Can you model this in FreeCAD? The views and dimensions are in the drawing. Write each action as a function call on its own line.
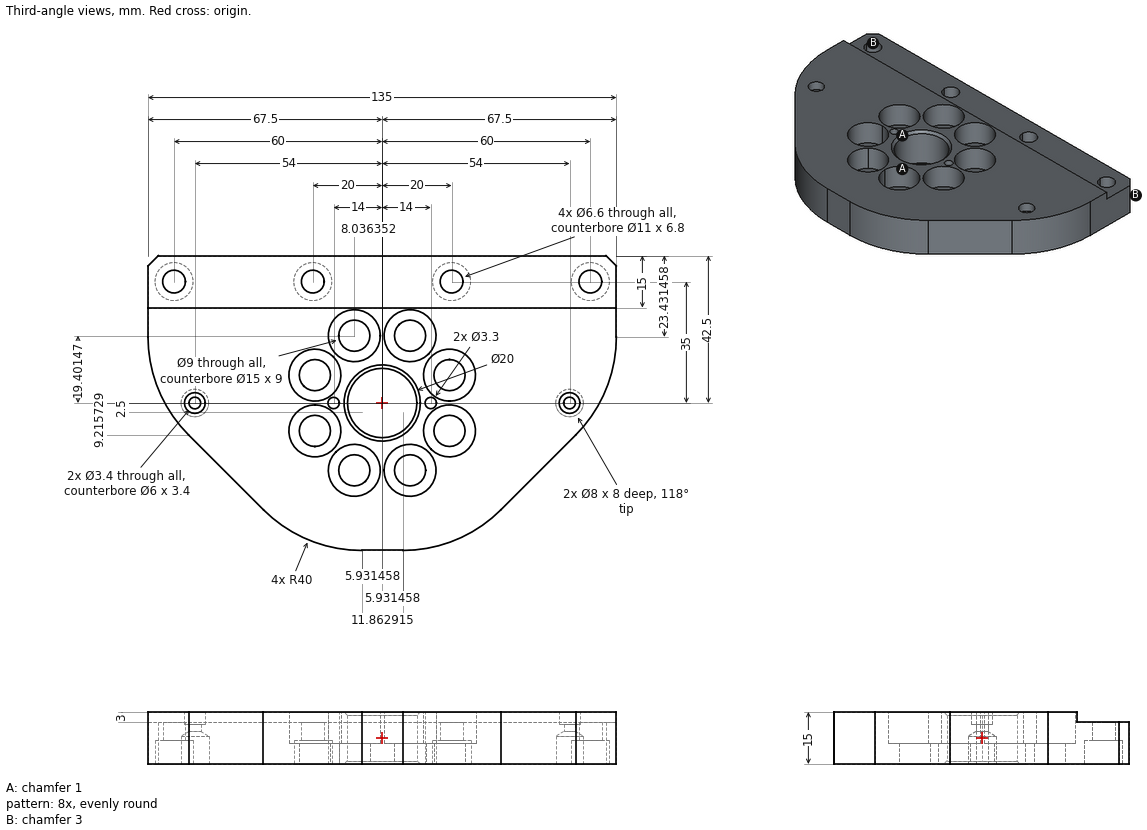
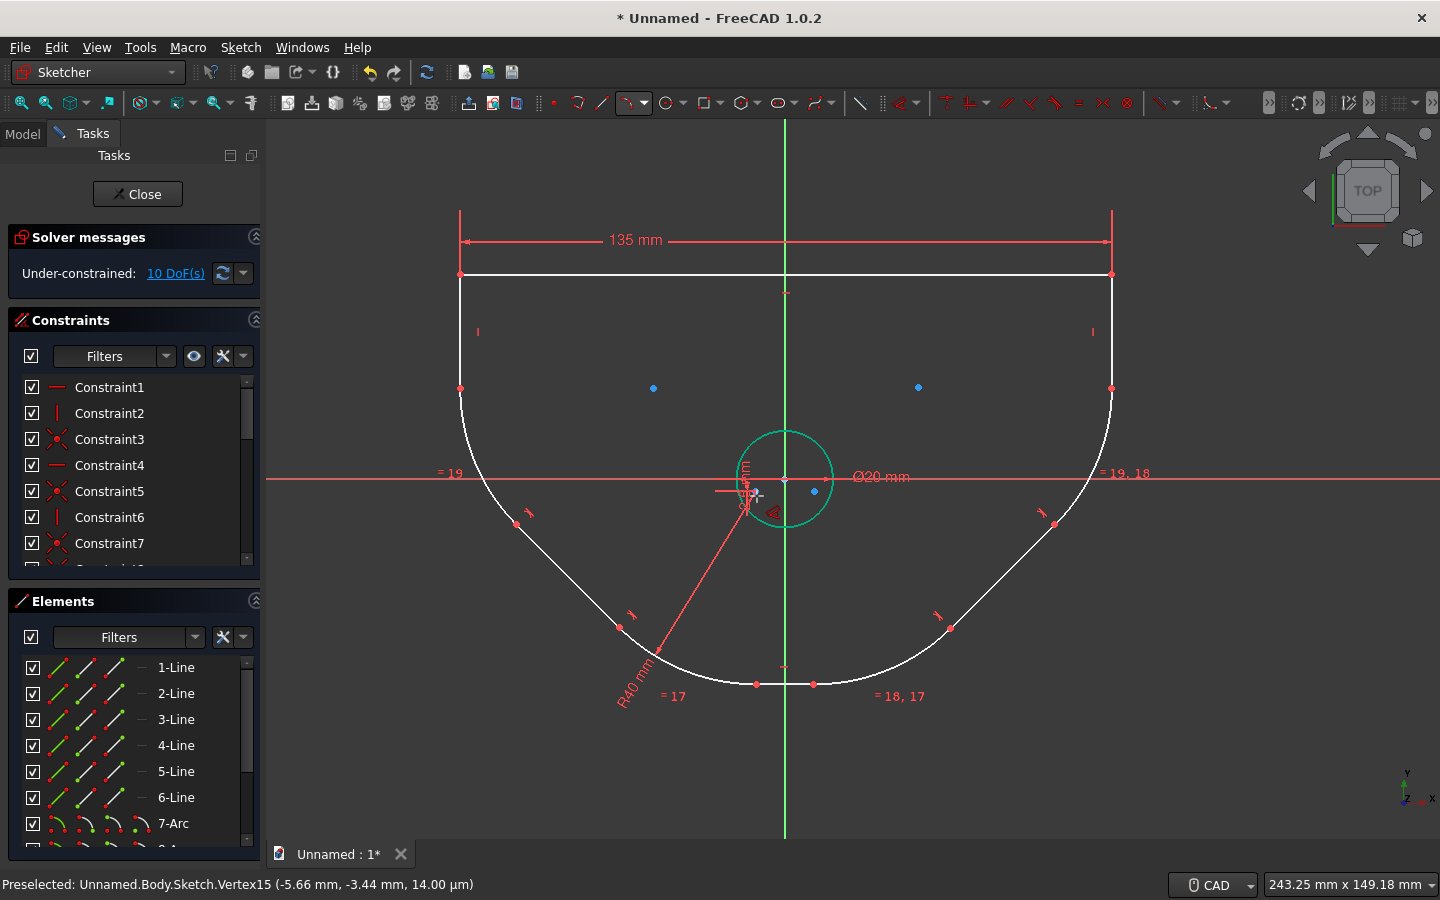
click(1112, 388)
click(948, 354)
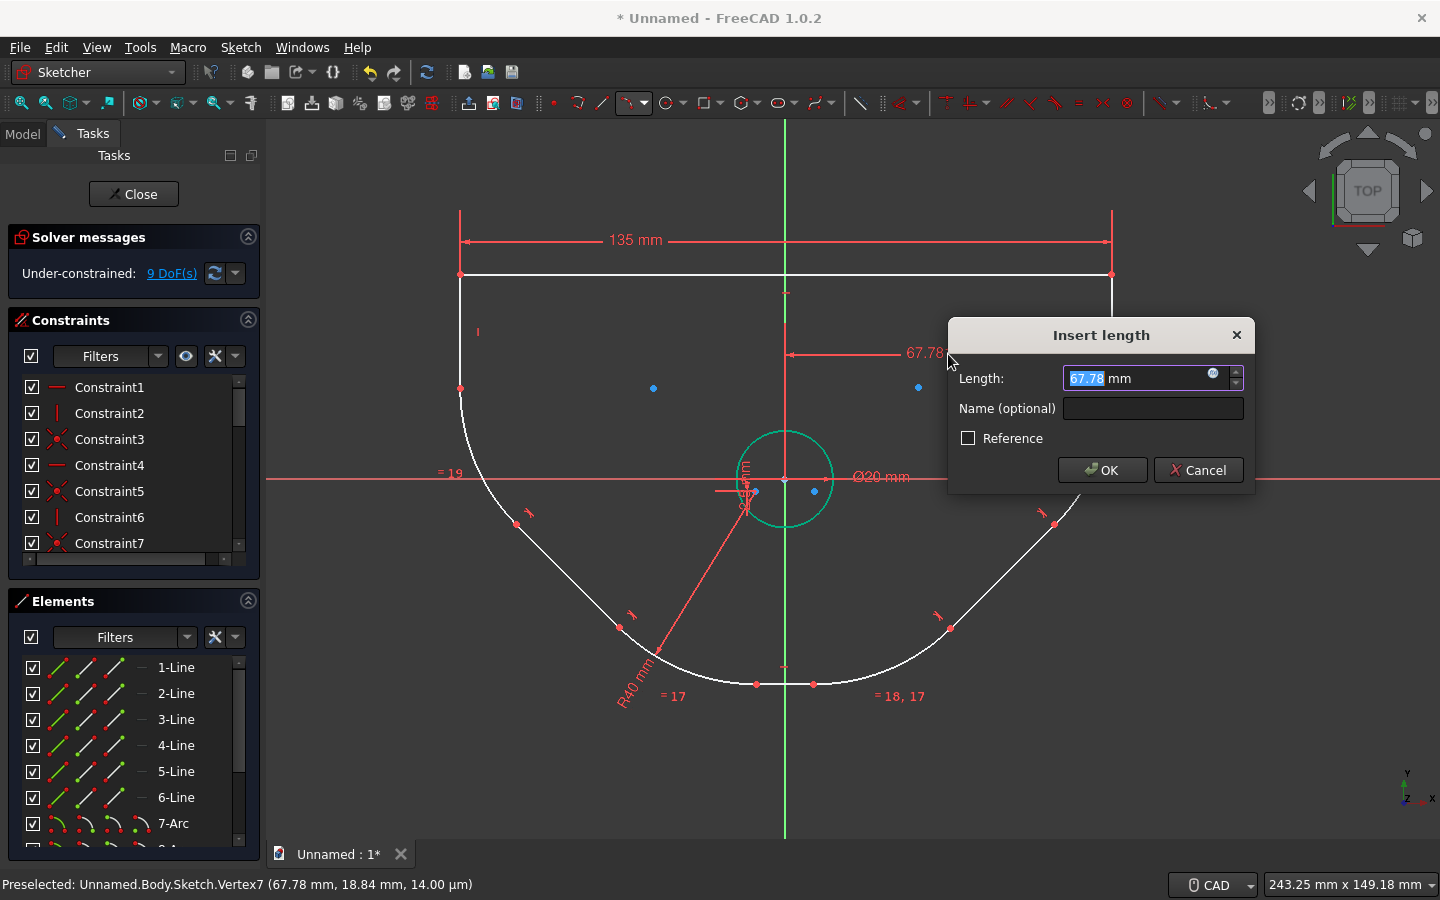
text(67.5)
key(Return)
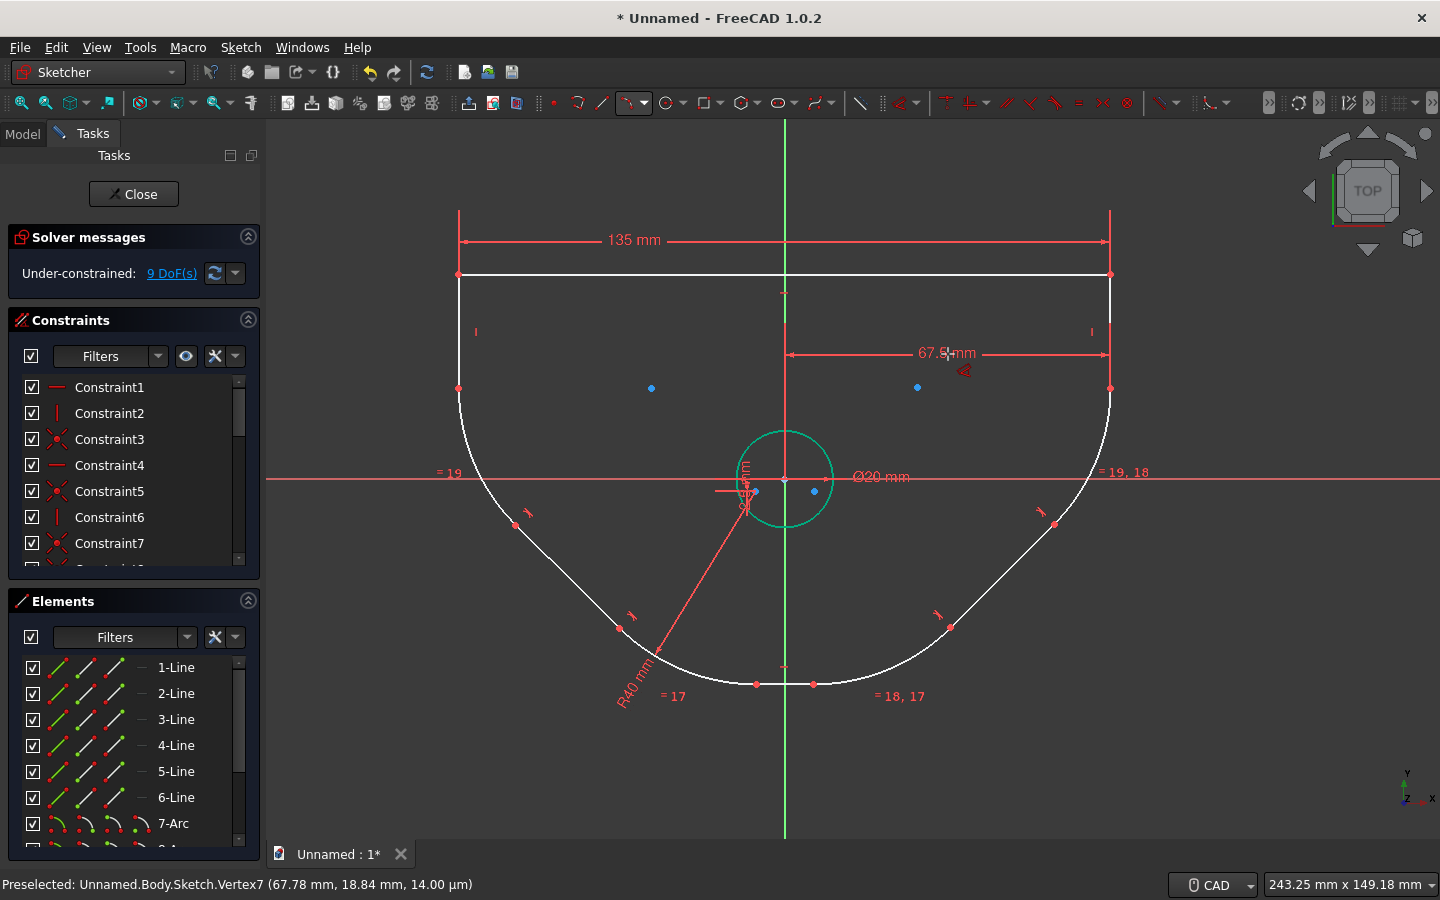
click(1110, 275)
click(1144, 377)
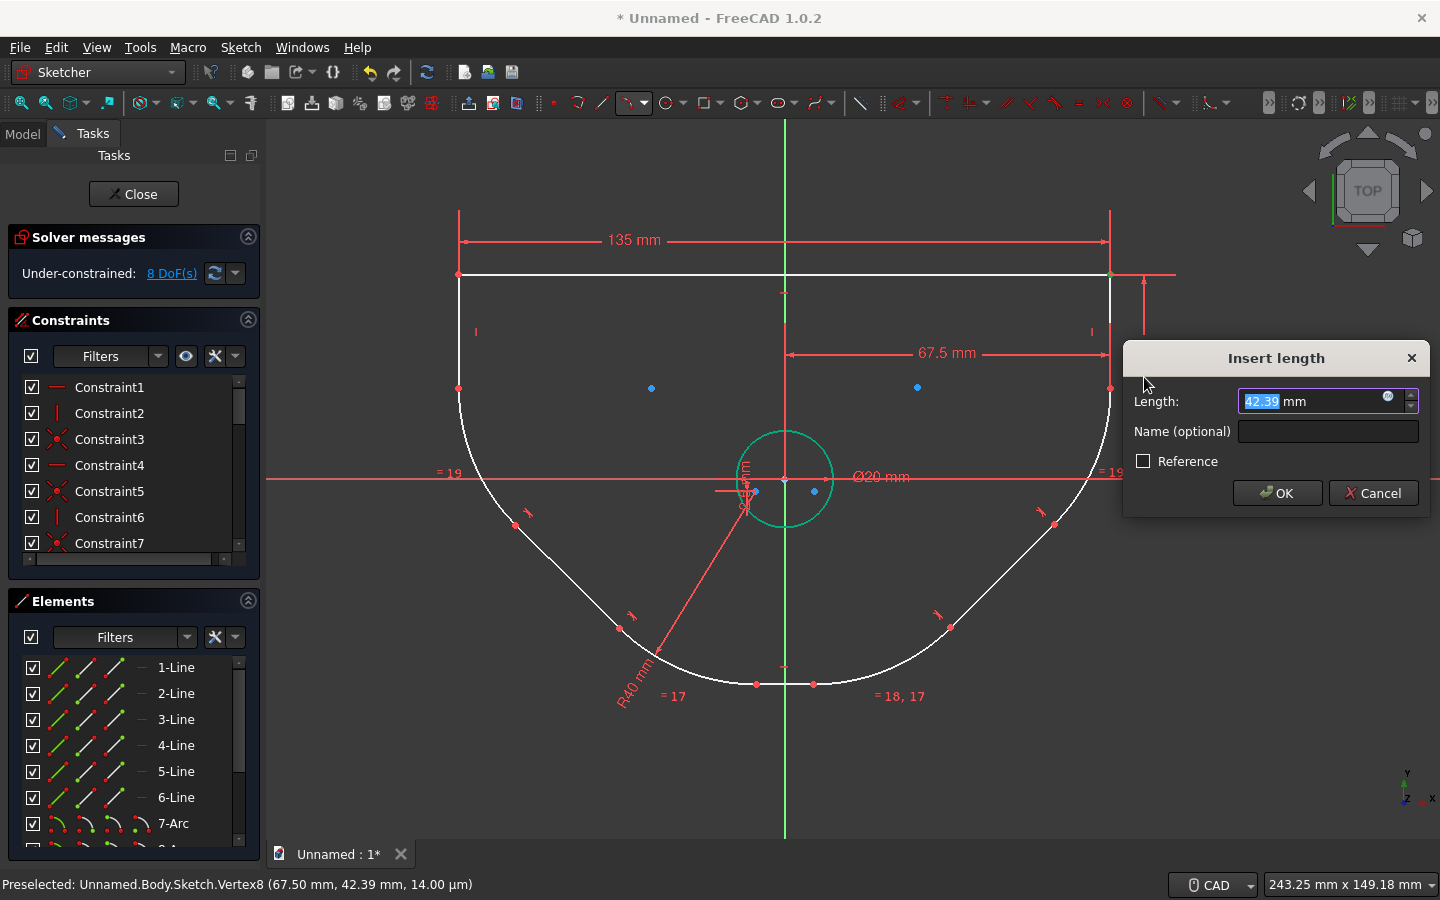
text(42.5)
key(Return)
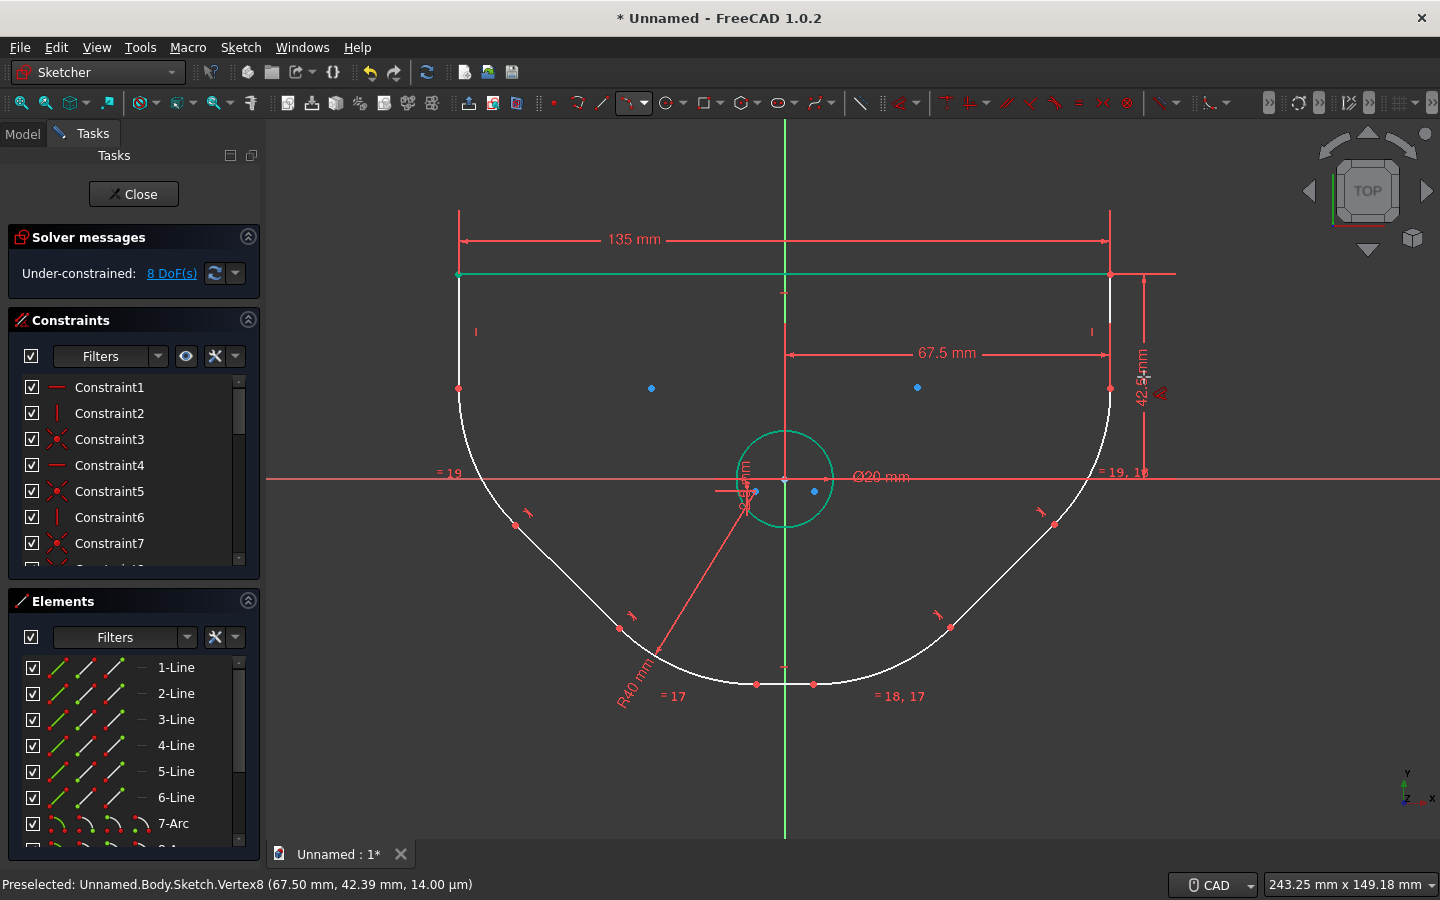
click(773, 684)
click(772, 718)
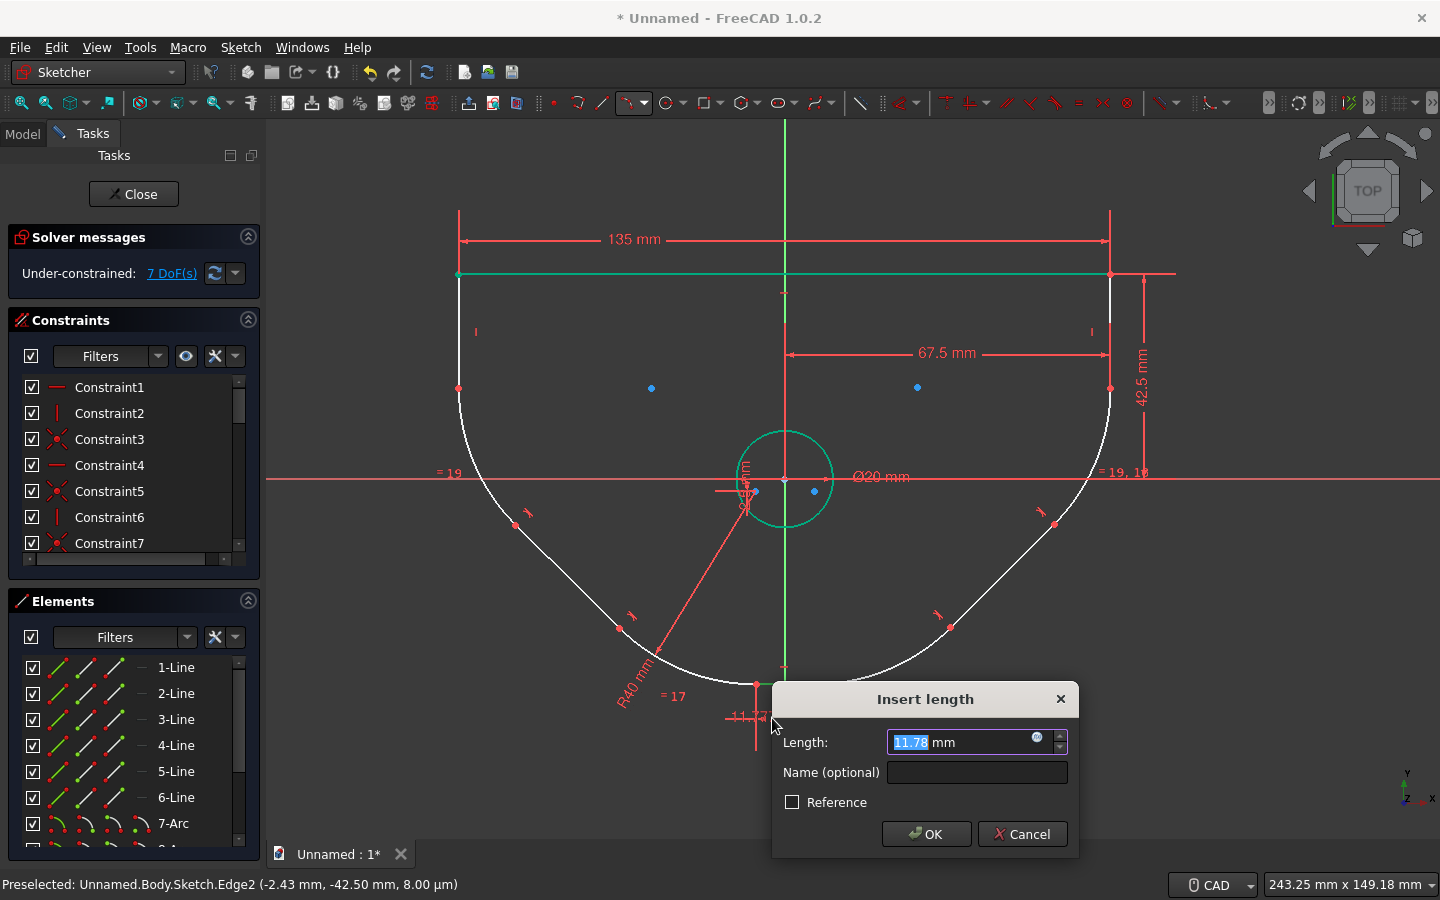
text(11.862915)
key(Return)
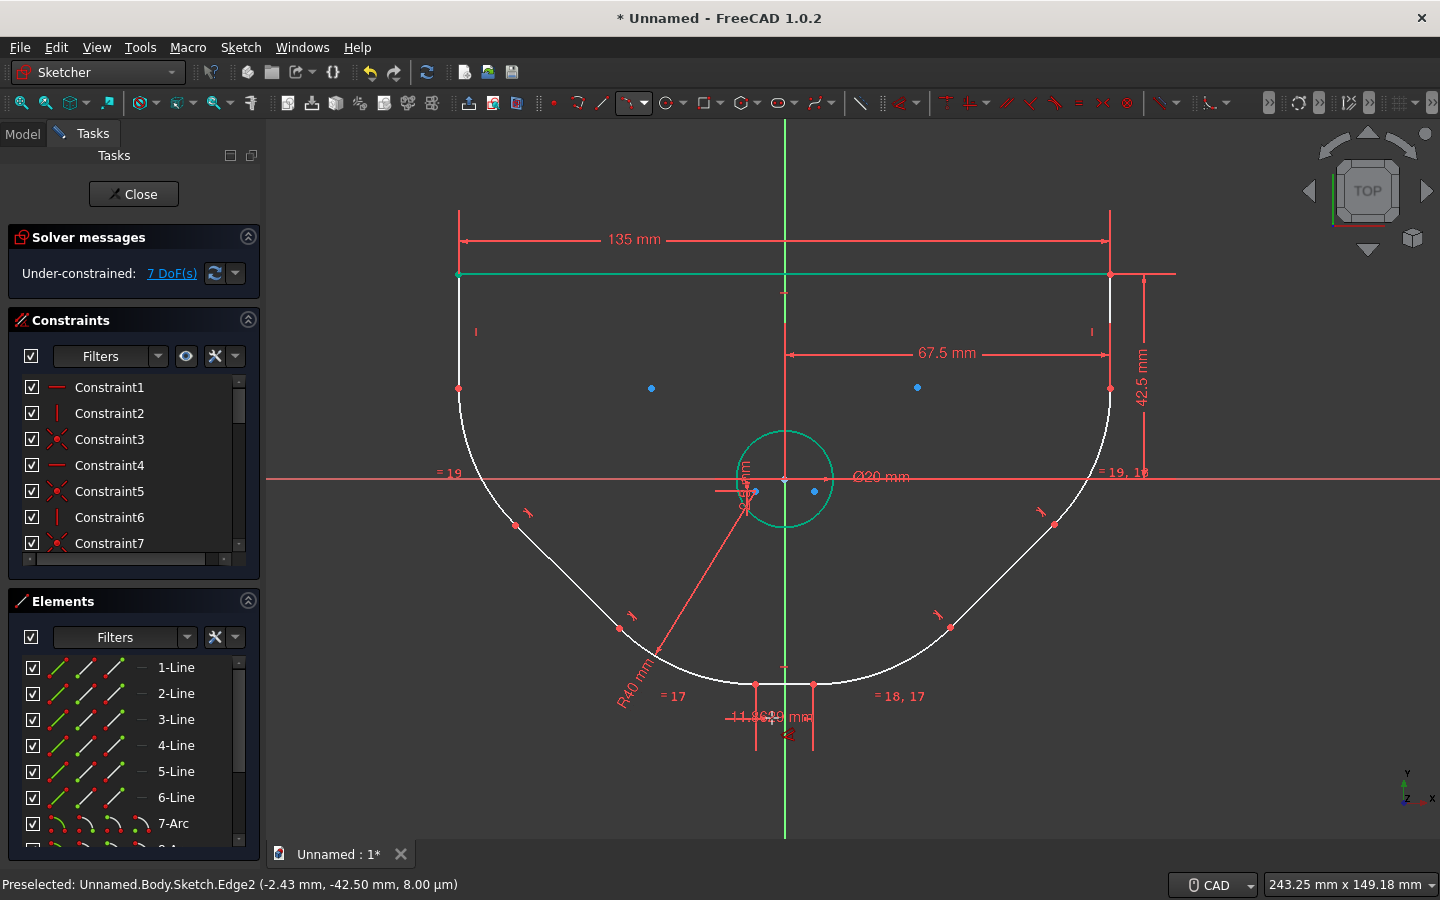
click(1110, 354)
click(1144, 331)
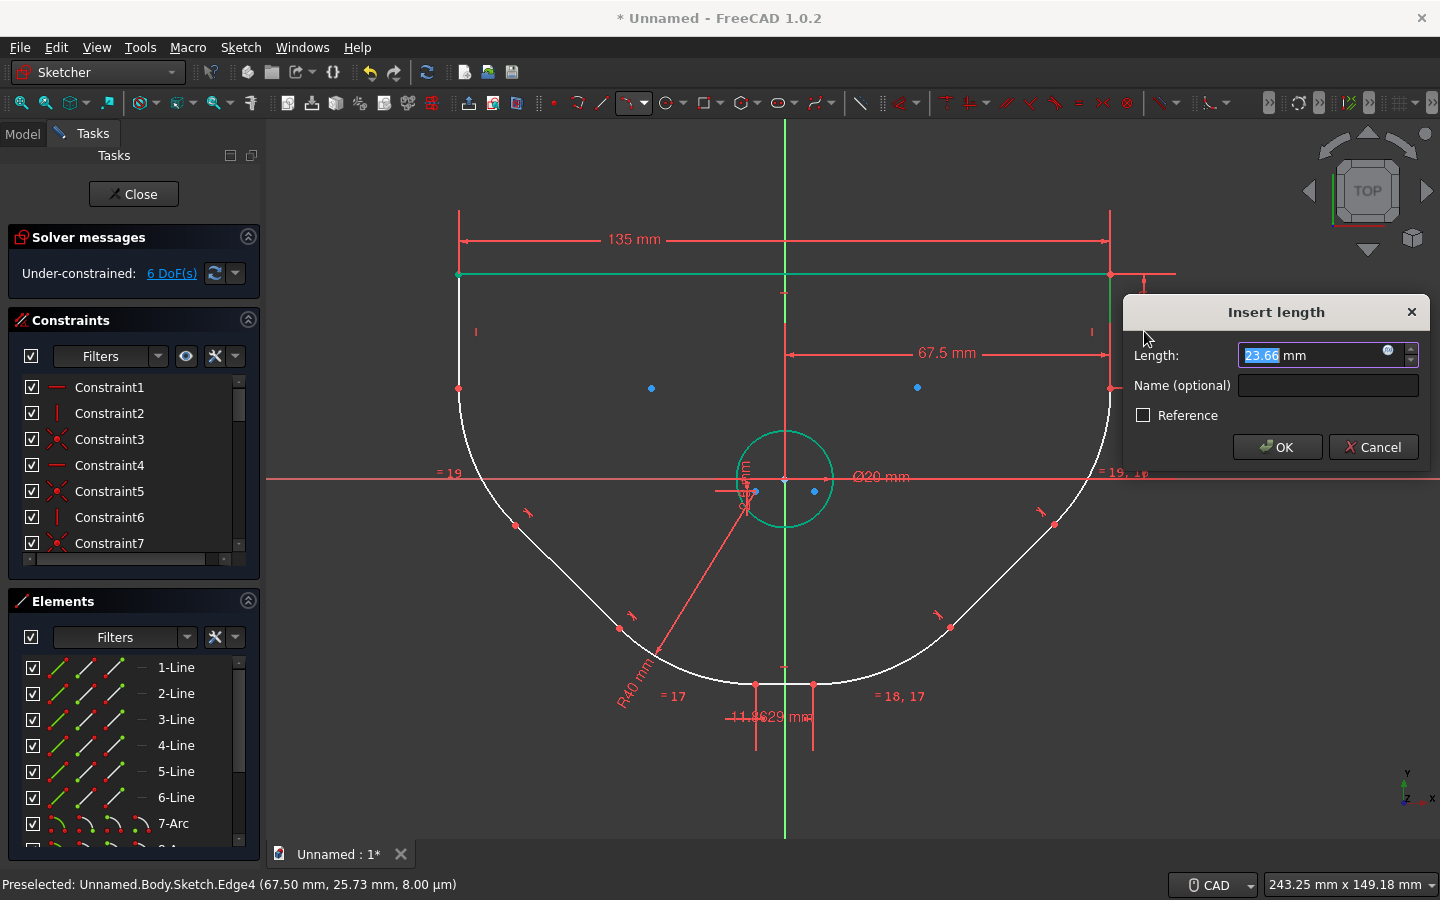
text(23.431458)
key(Return)